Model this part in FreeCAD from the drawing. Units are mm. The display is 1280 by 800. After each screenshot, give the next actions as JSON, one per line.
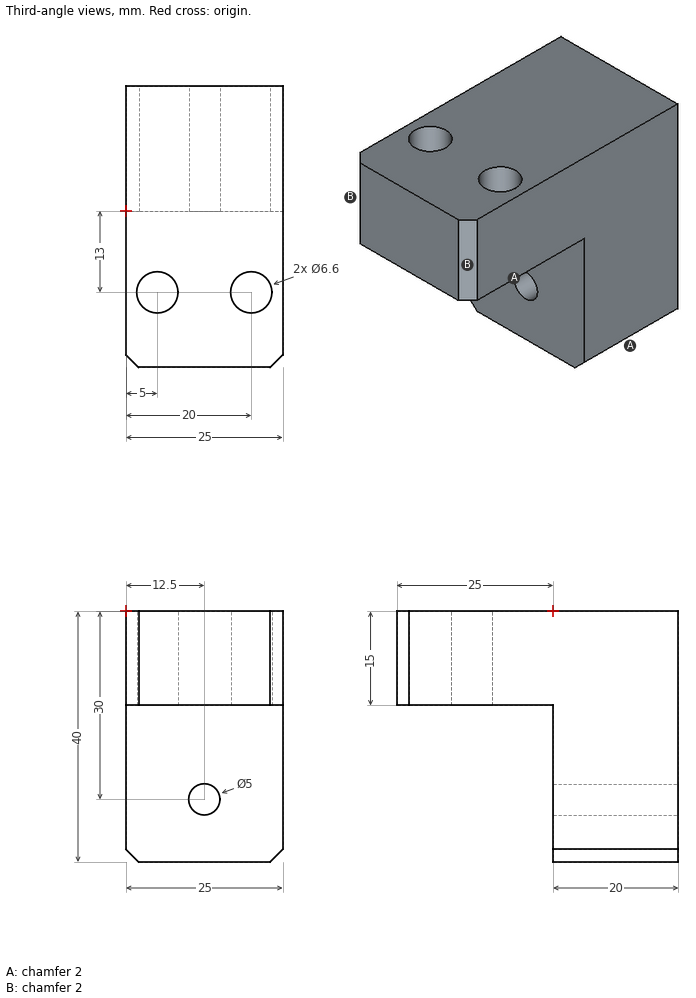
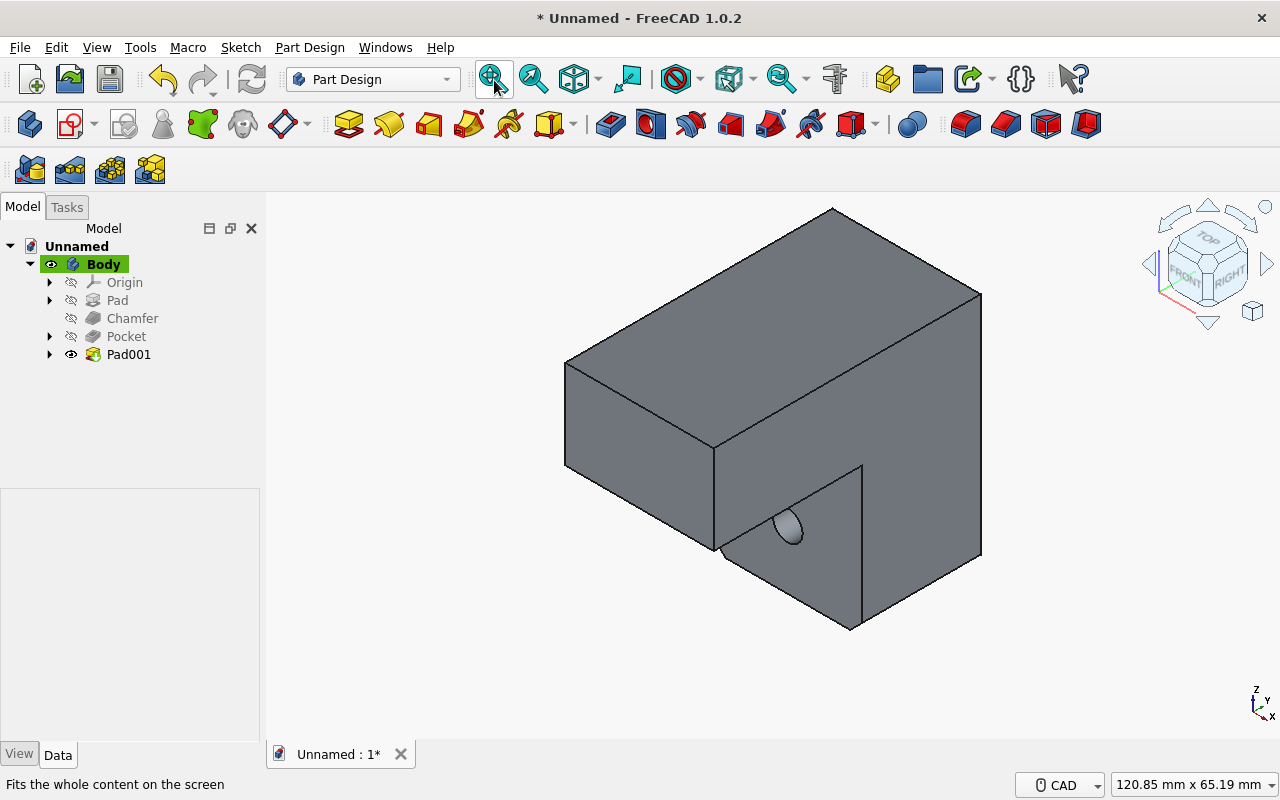
{"action": "key", "text": "5"}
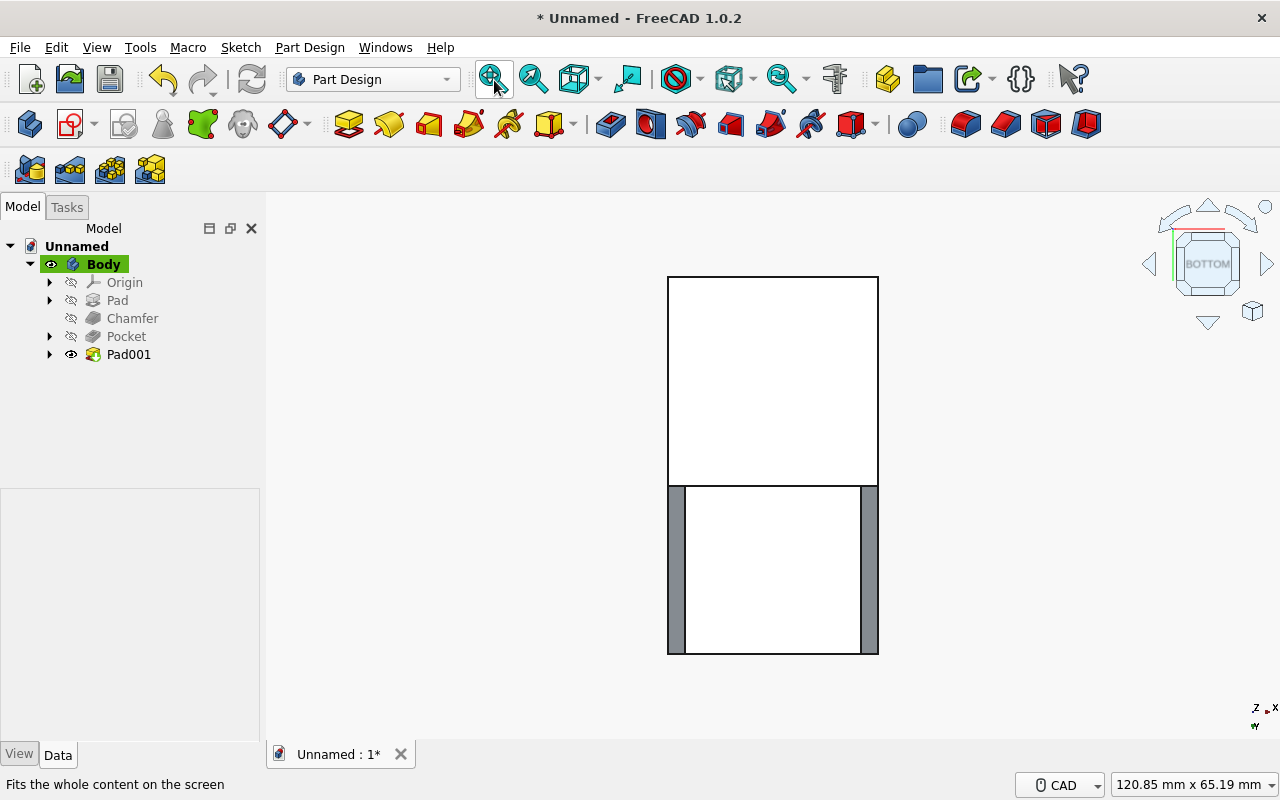
{"action": "left_click", "coordinate": [773, 381]}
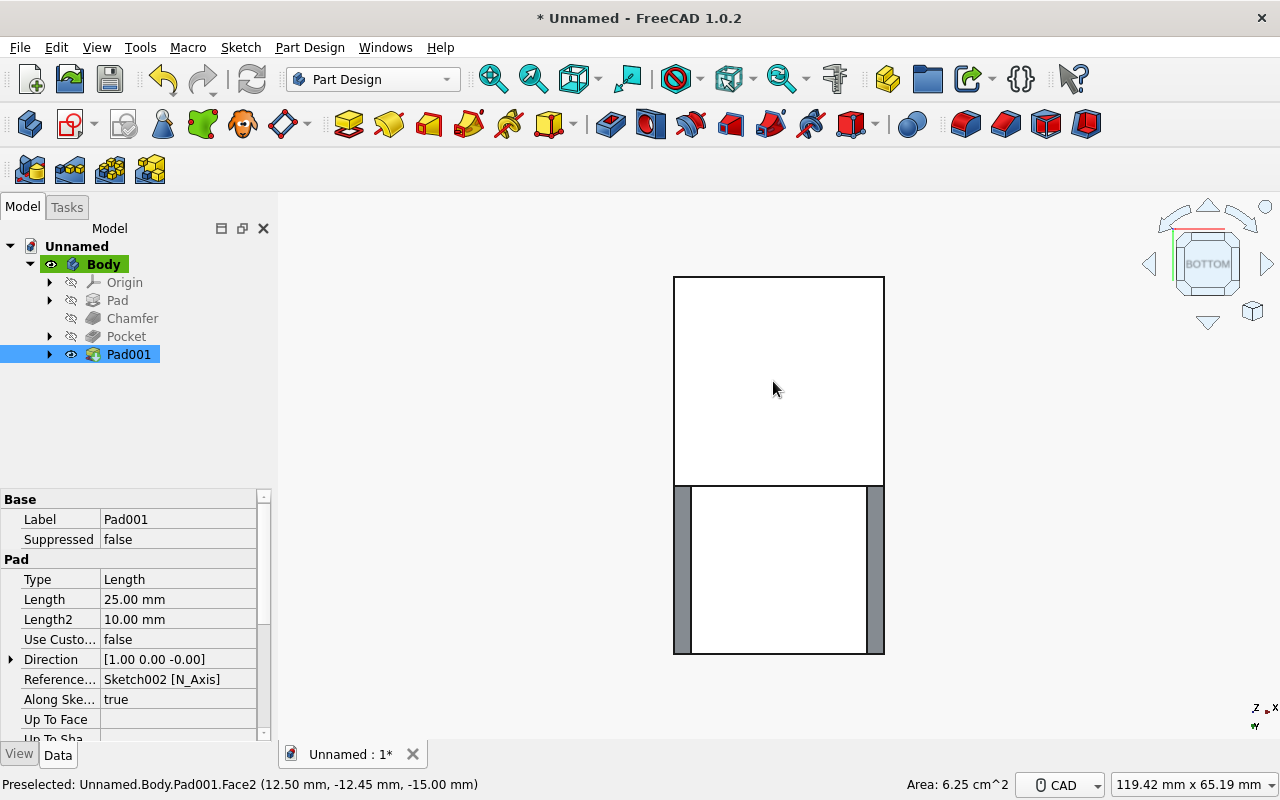
{"action": "left_click", "coordinate": [70, 124]}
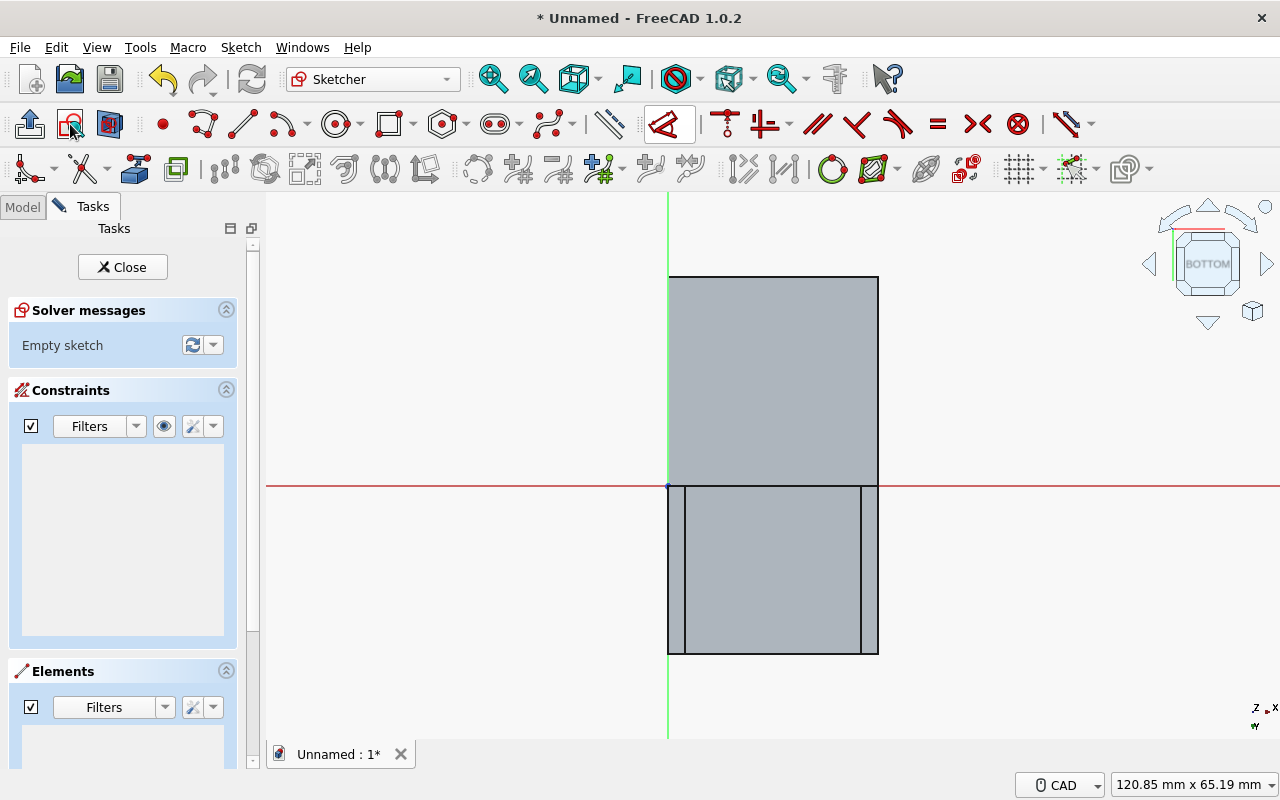
{"action": "key", "text": "q s"}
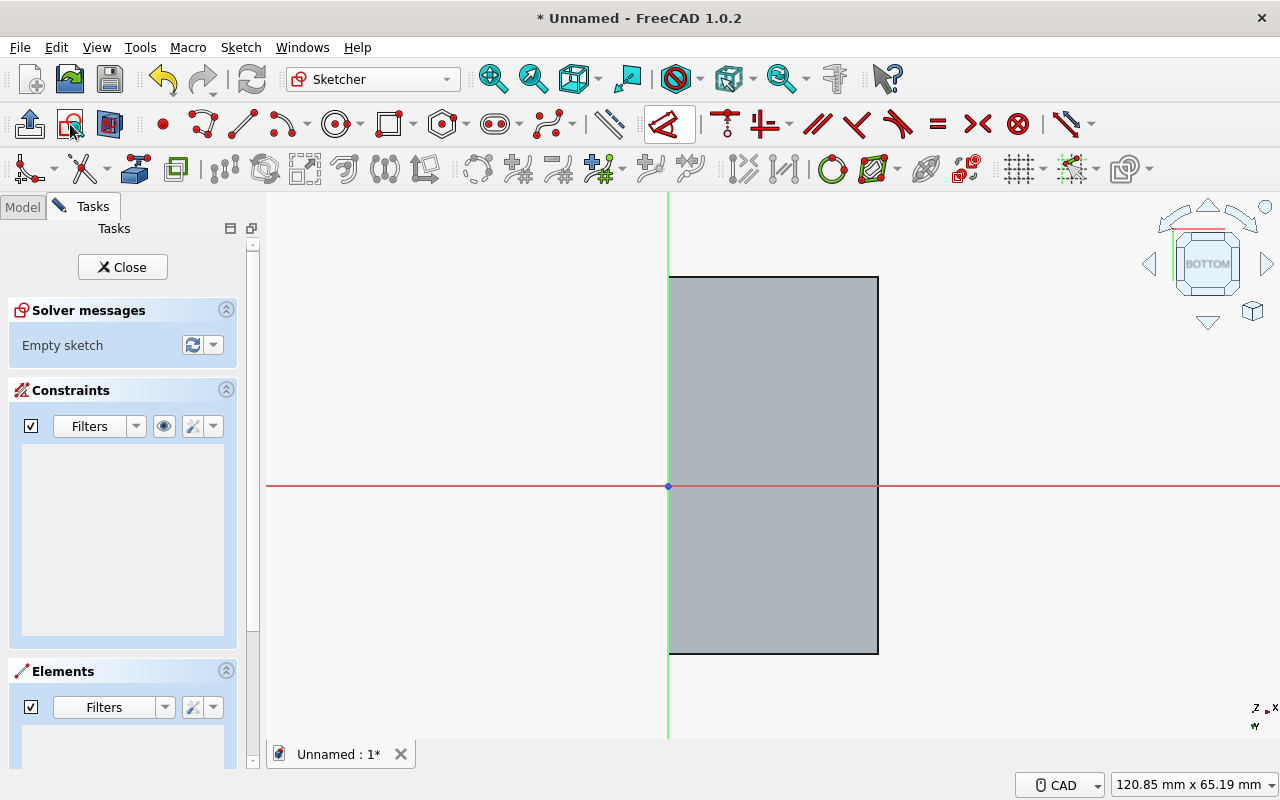
{"action": "scroll", "coordinate": [802, 391], "scroll_direction": "up", "scroll_amount": 5}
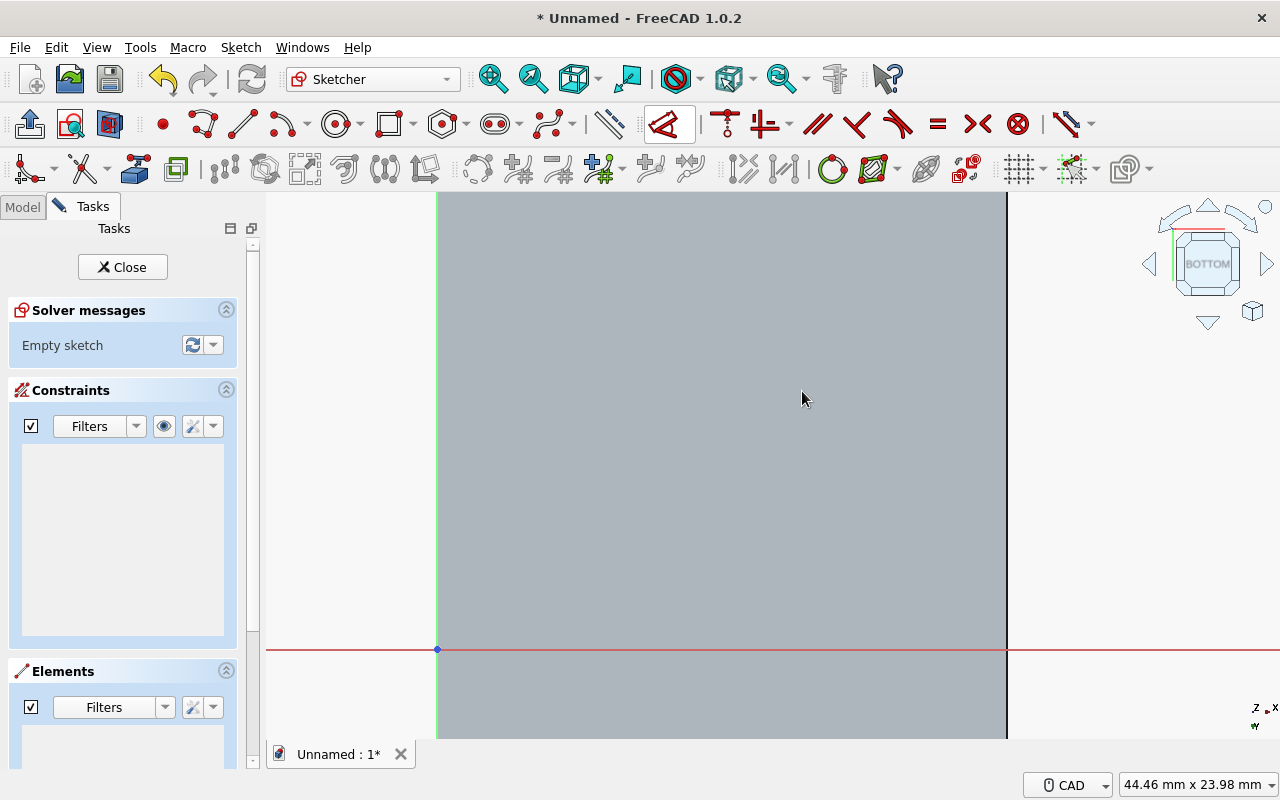
{"action": "left_click", "coordinate": [336, 124]}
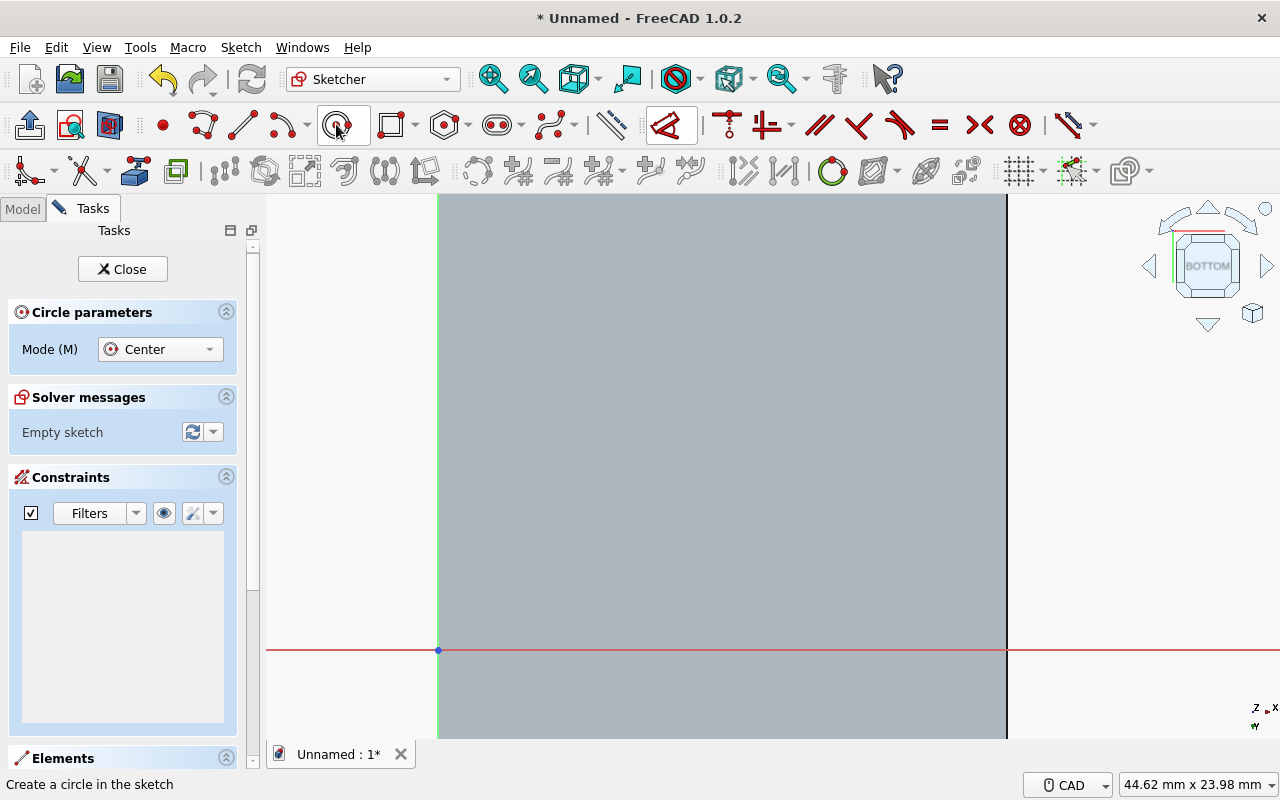
{"action": "left_click", "coordinate": [893, 355]}
{"action": "left_click", "coordinate": [946, 302]}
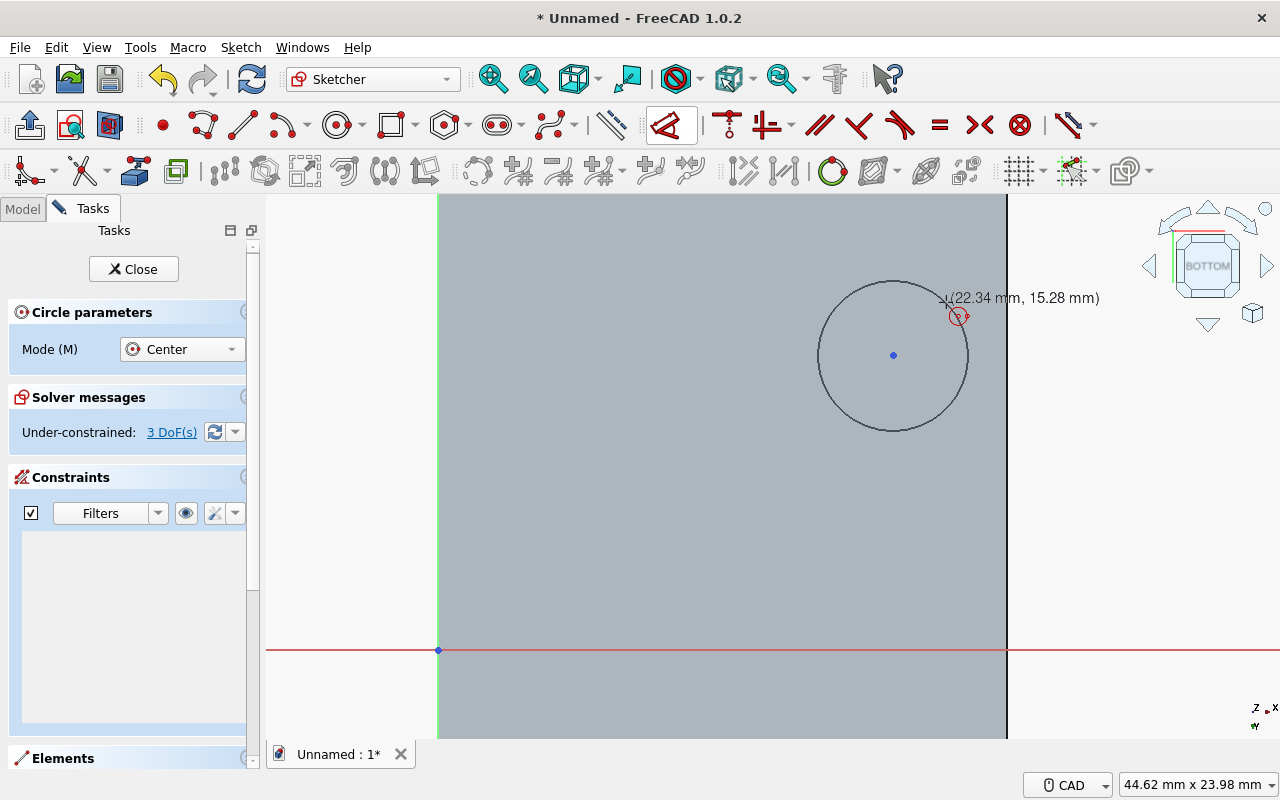
{"action": "left_click", "coordinate": [552, 355]}
{"action": "left_click", "coordinate": [605, 302]}
{"action": "key", "text": "Escape"}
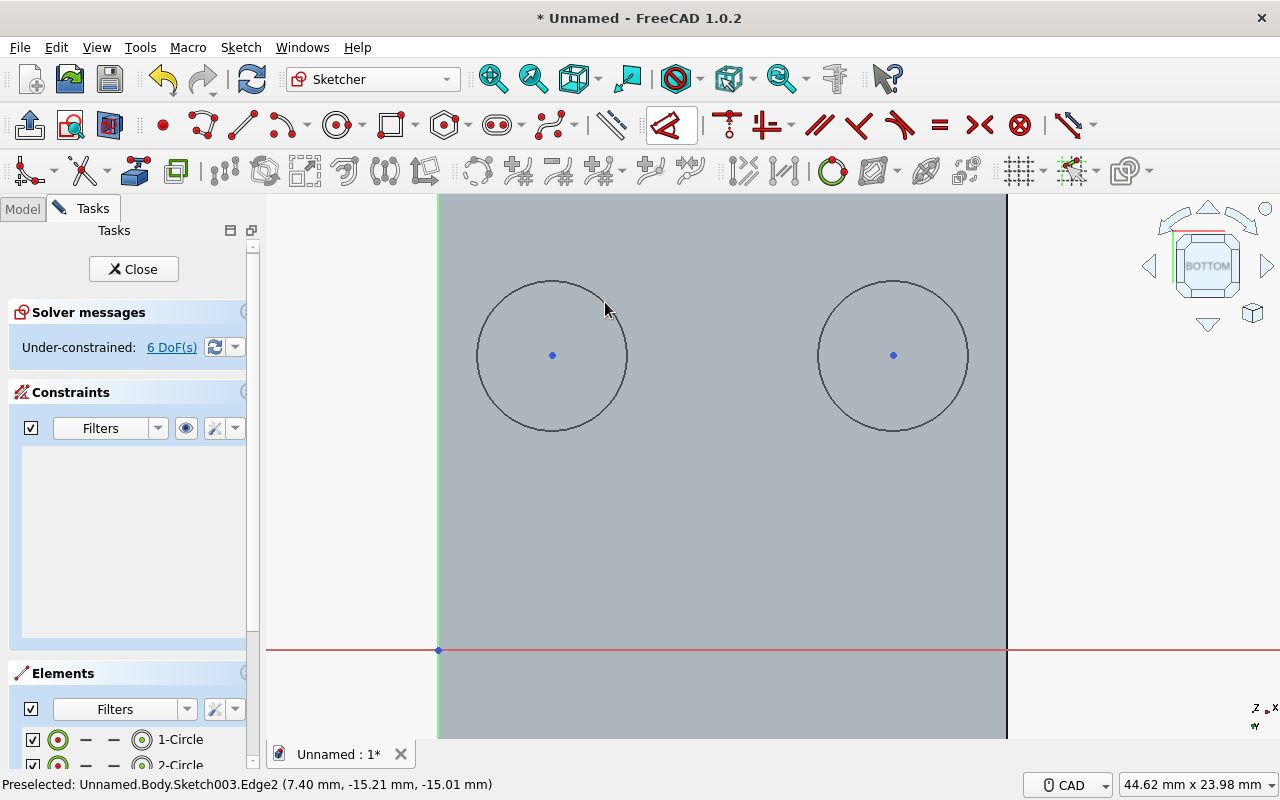
{"action": "left_click", "coordinate": [946, 303]}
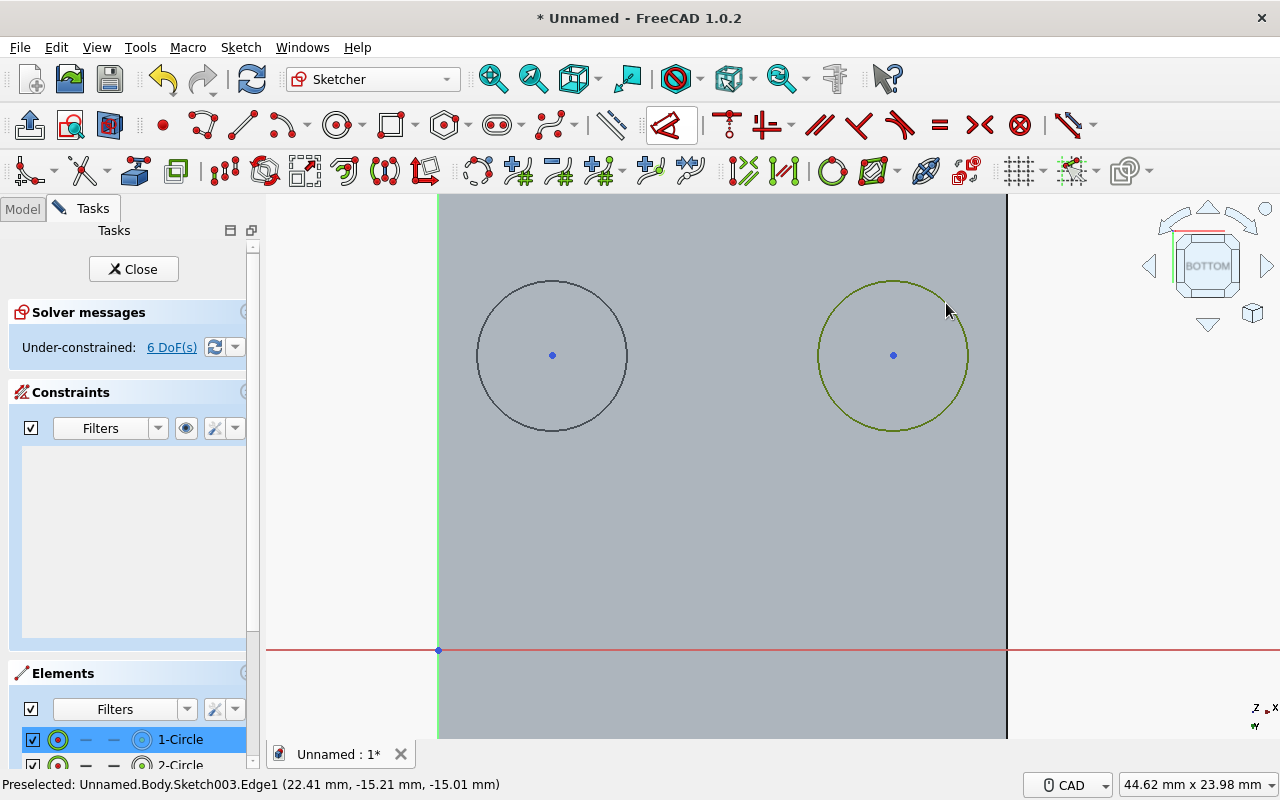
{"action": "left_click", "coordinate": [605, 303]}